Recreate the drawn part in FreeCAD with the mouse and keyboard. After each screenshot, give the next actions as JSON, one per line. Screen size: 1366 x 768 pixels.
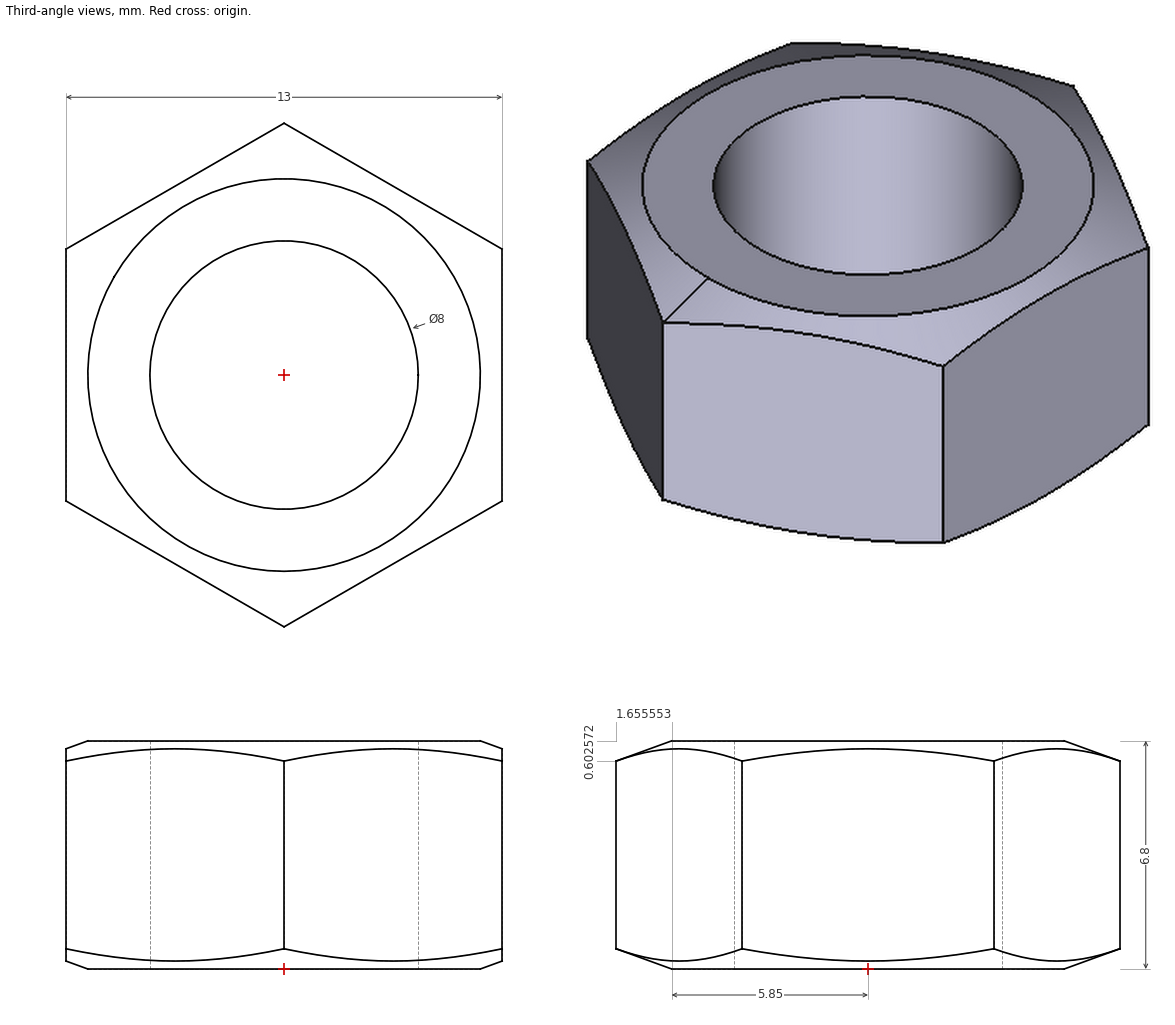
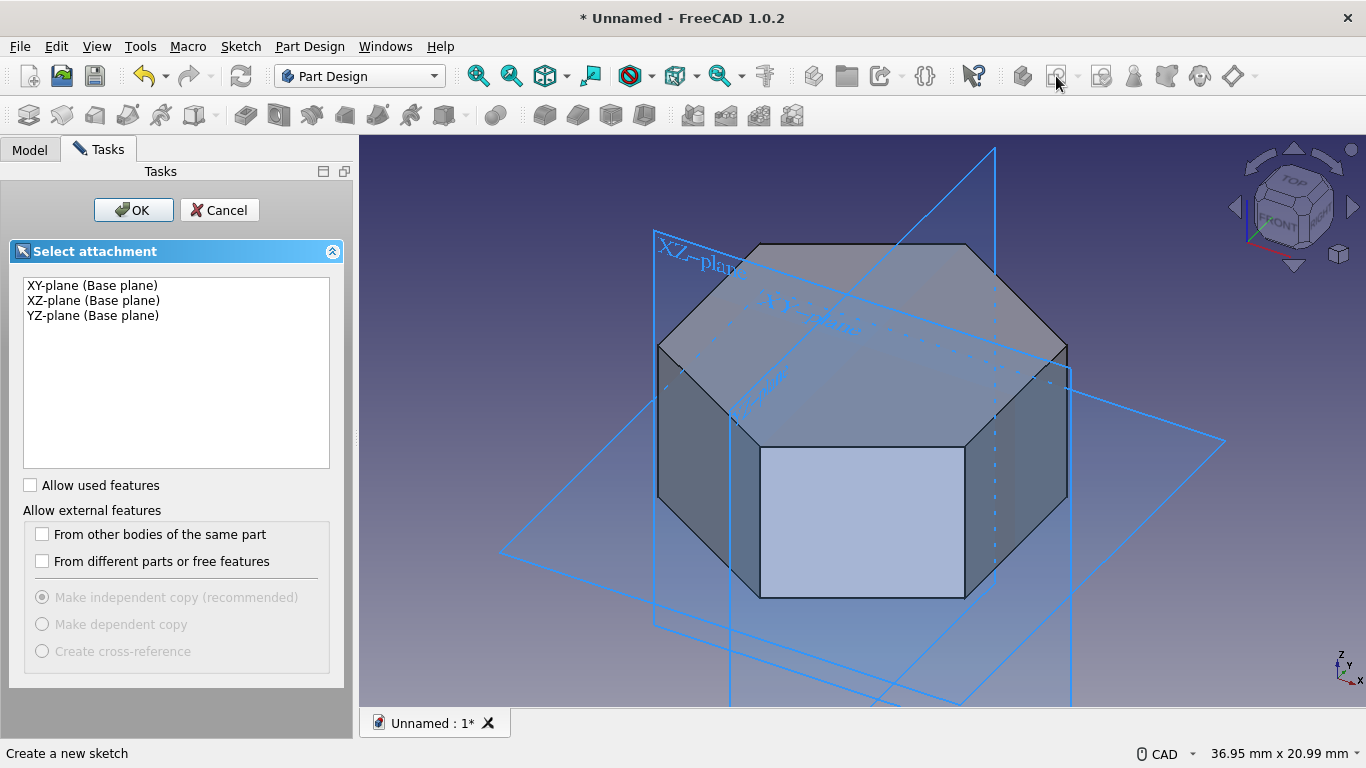
{"action": "left_click", "coordinate": [84, 316]}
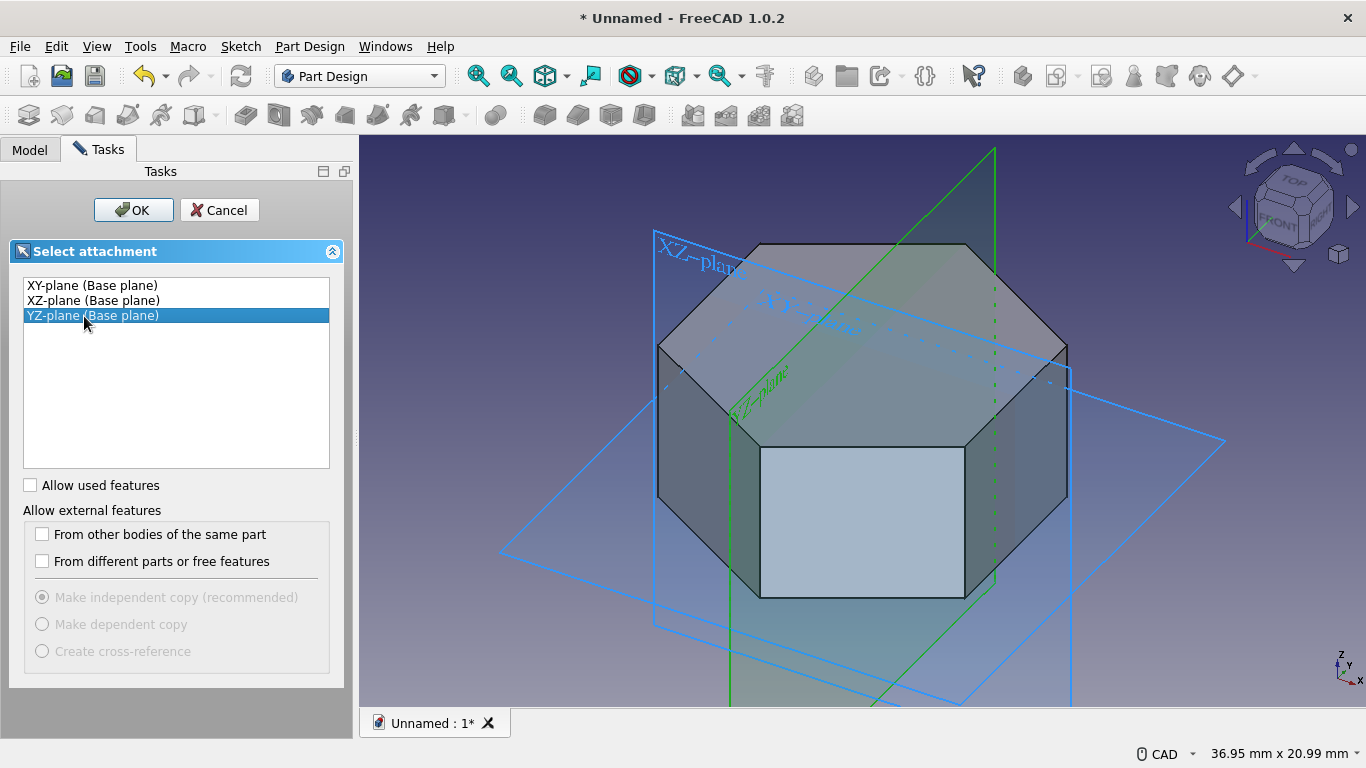
{"action": "left_click", "coordinate": [134, 210]}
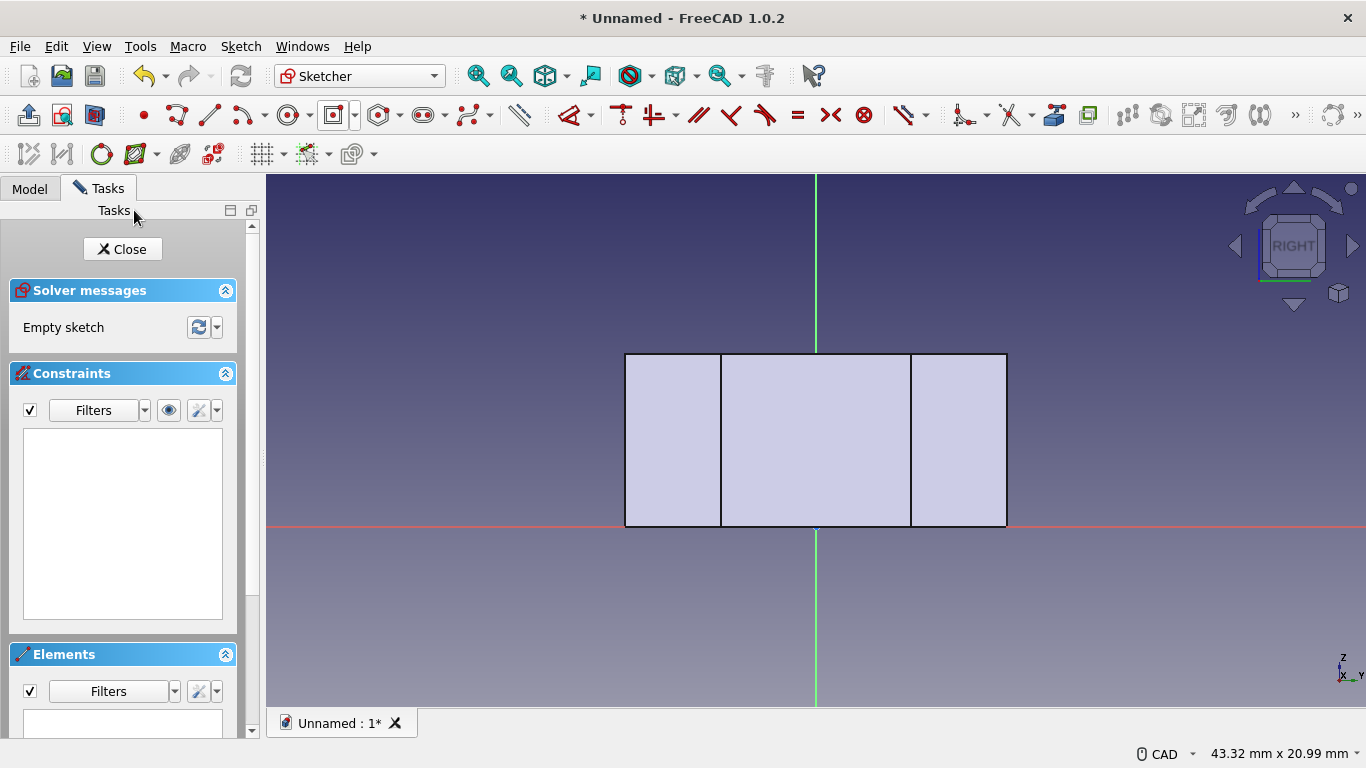
{"action": "key", "text": "q s"}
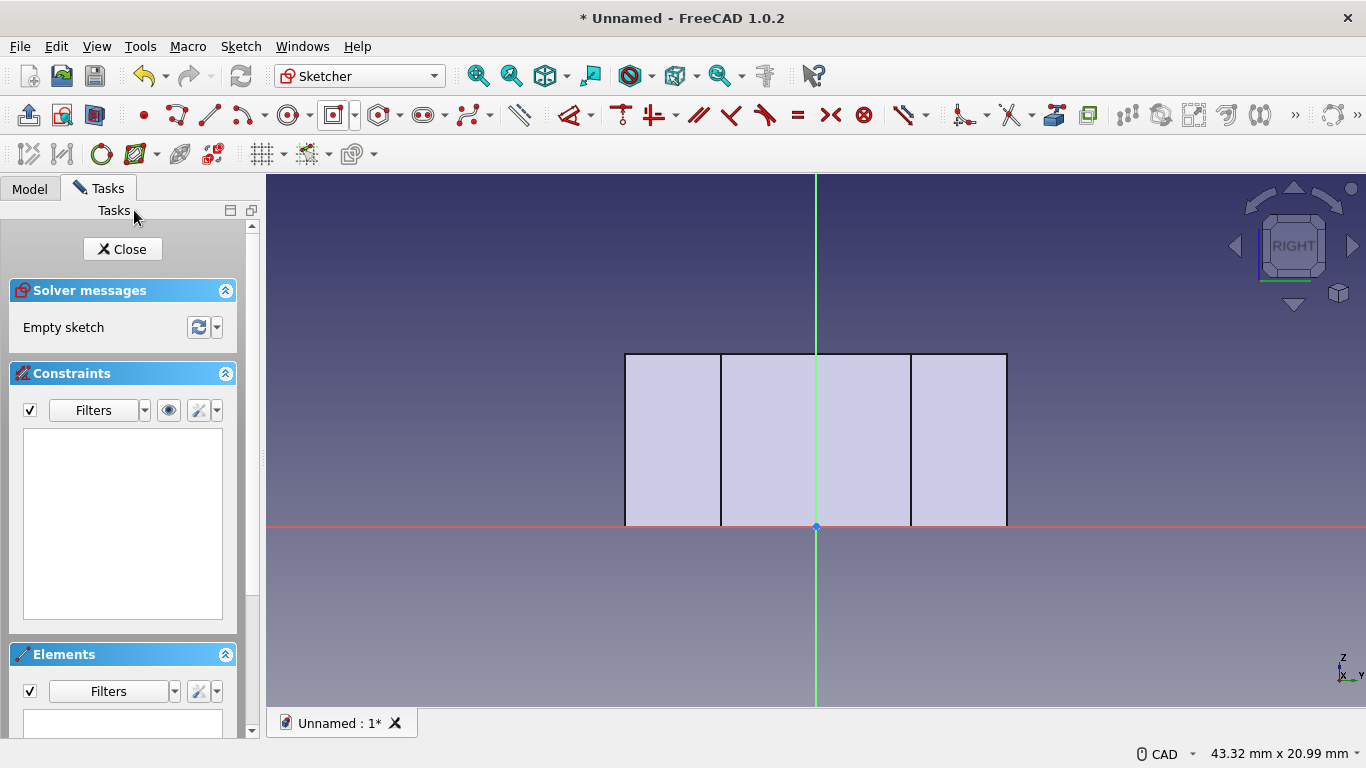
{"action": "scroll", "coordinate": [640, 357], "scroll_direction": "up", "scroll_amount": 14}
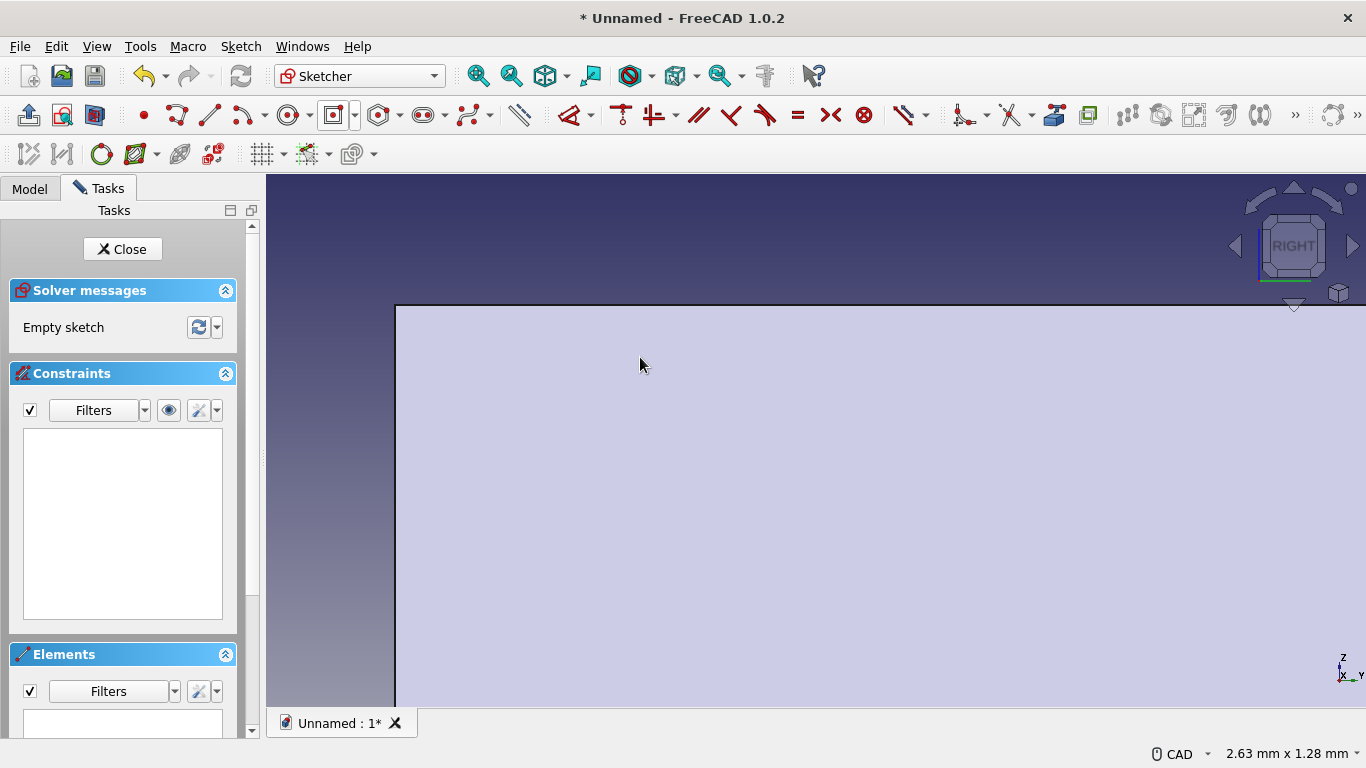
{"action": "key", "text": "g m"}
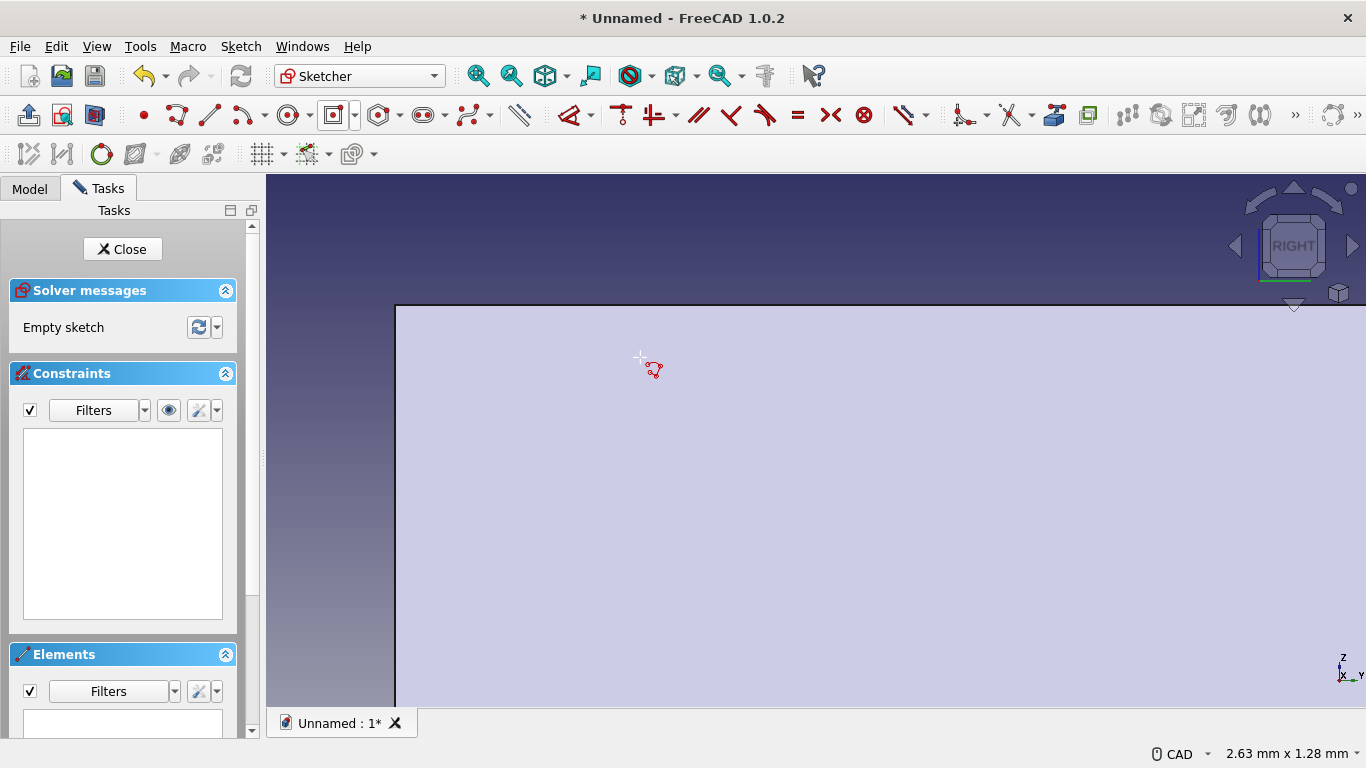
{"action": "left_click", "coordinate": [1086, 305]}
{"action": "left_click", "coordinate": [395, 305]}
{"action": "left_click", "coordinate": [395, 557]}
{"action": "left_click", "coordinate": [1086, 306]}
{"action": "key", "text": "Escape"}
{"action": "key", "text": "Escape"}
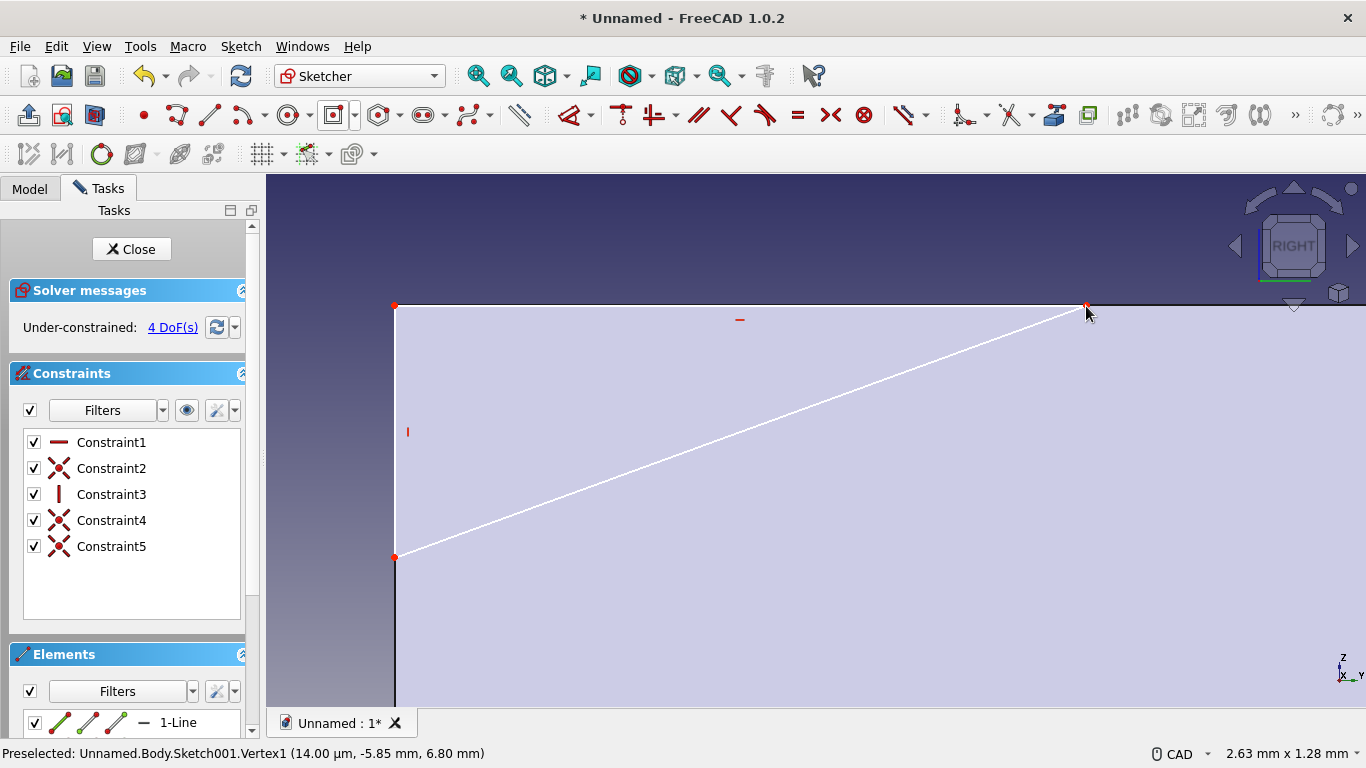
{"action": "key", "text": "d"}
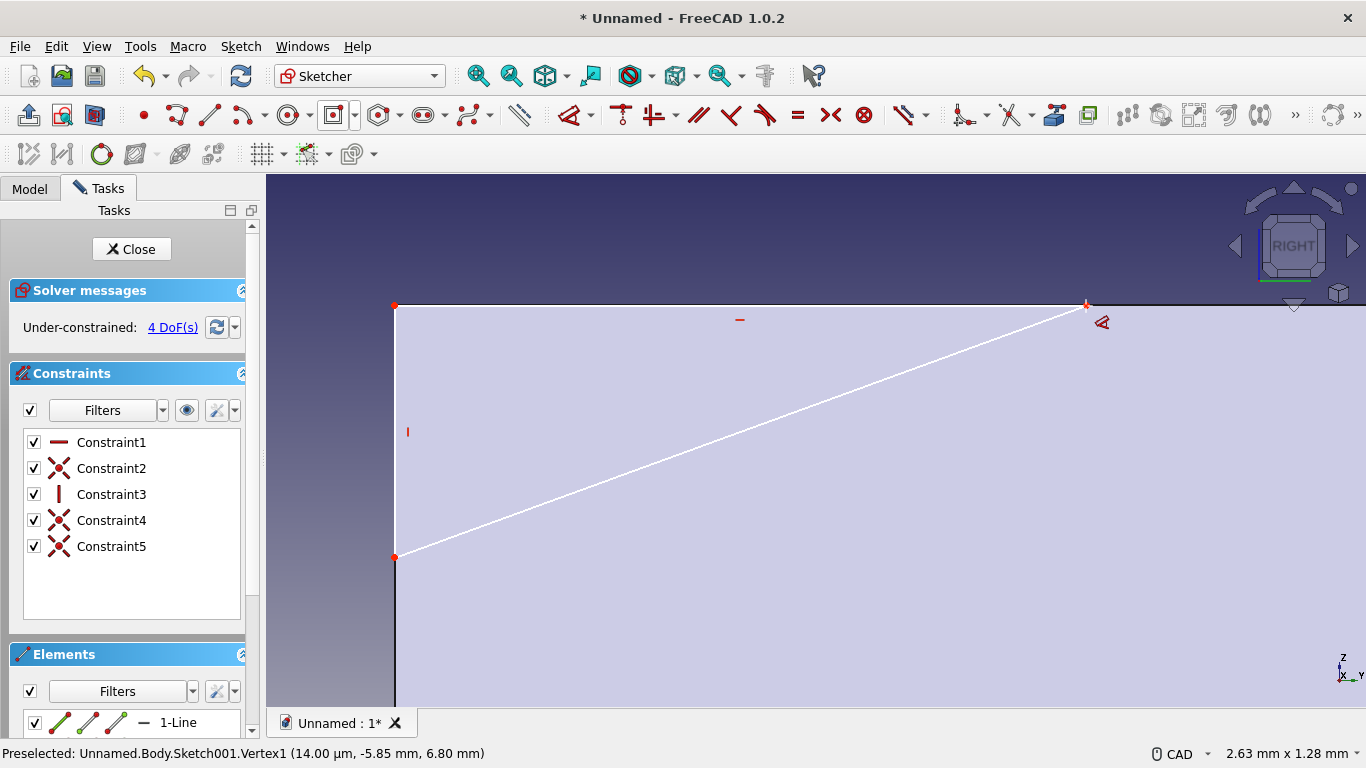
{"action": "left_click", "coordinate": [1086, 306]}
{"action": "left_click", "coordinate": [1052, 492]}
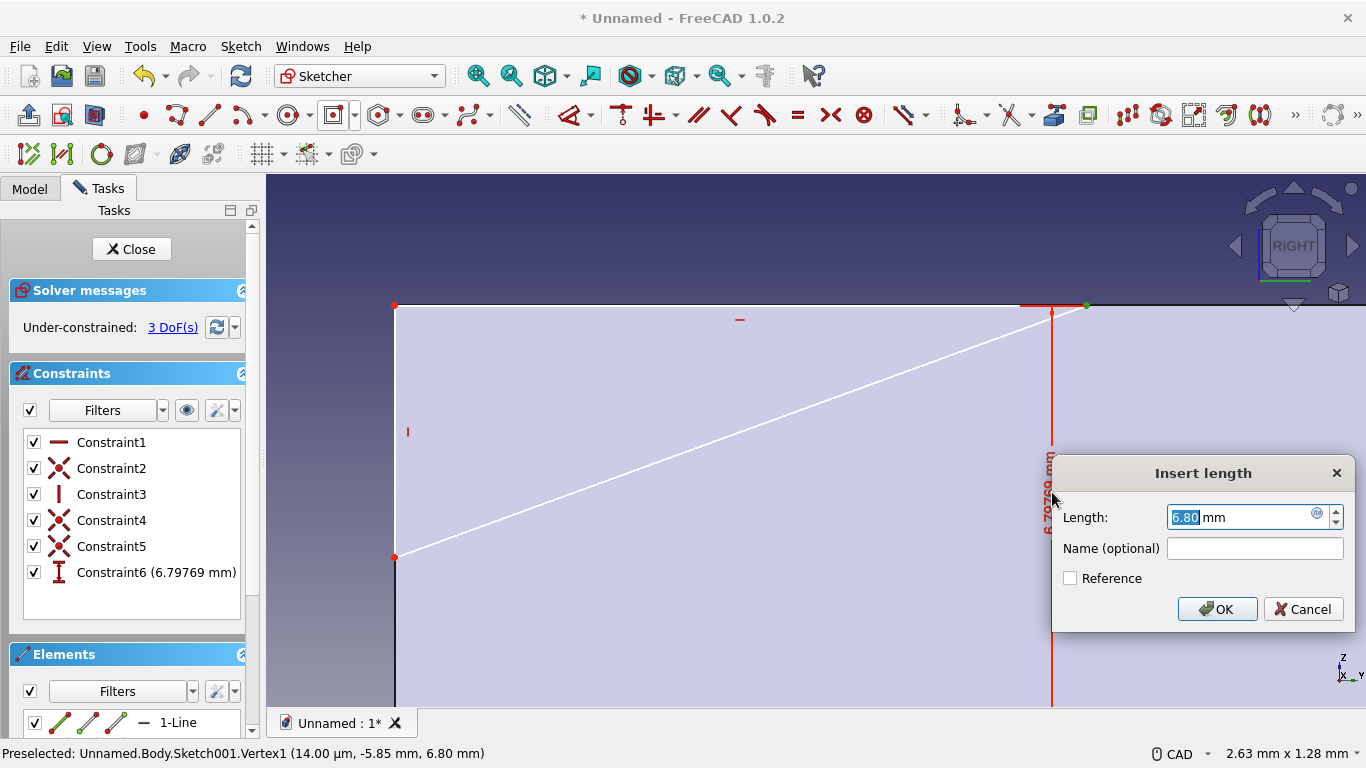
{"action": "type", "text": "6.8"}
{"action": "key", "text": "Return"}